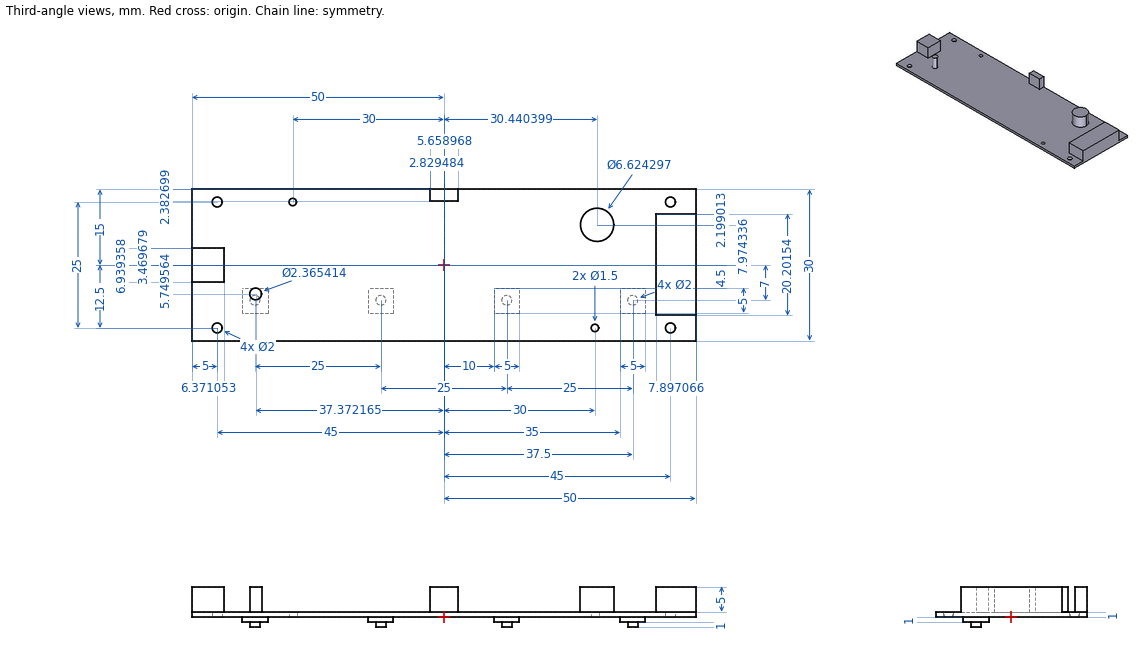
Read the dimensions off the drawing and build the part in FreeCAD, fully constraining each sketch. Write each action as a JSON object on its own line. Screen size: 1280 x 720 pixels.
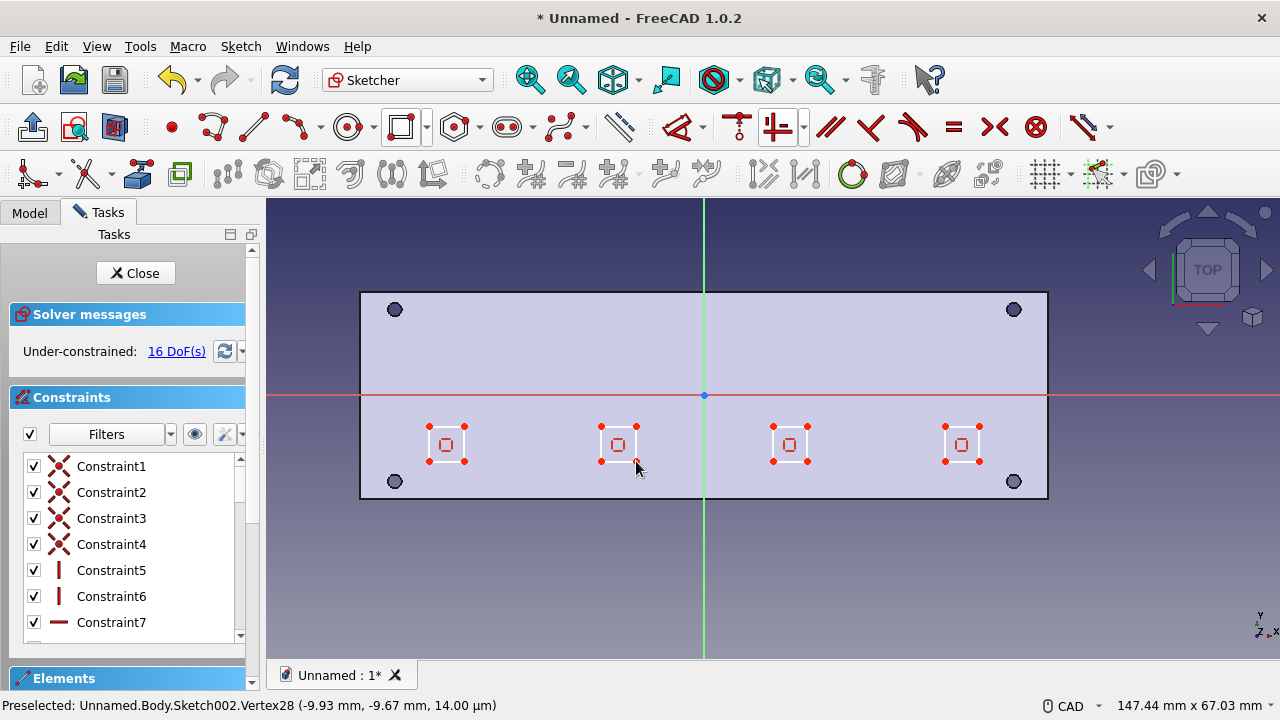
{"action": "left_click", "coordinate": [979, 427]}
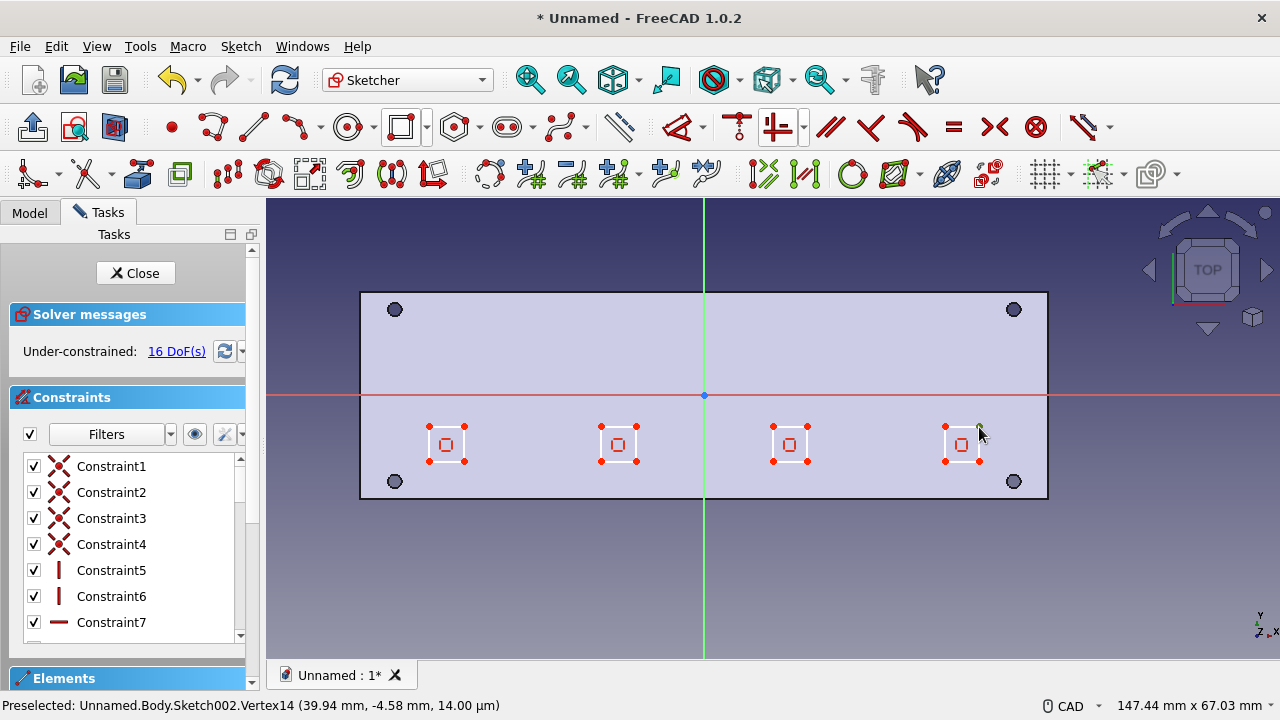
{"action": "left_click", "coordinate": [429, 427]}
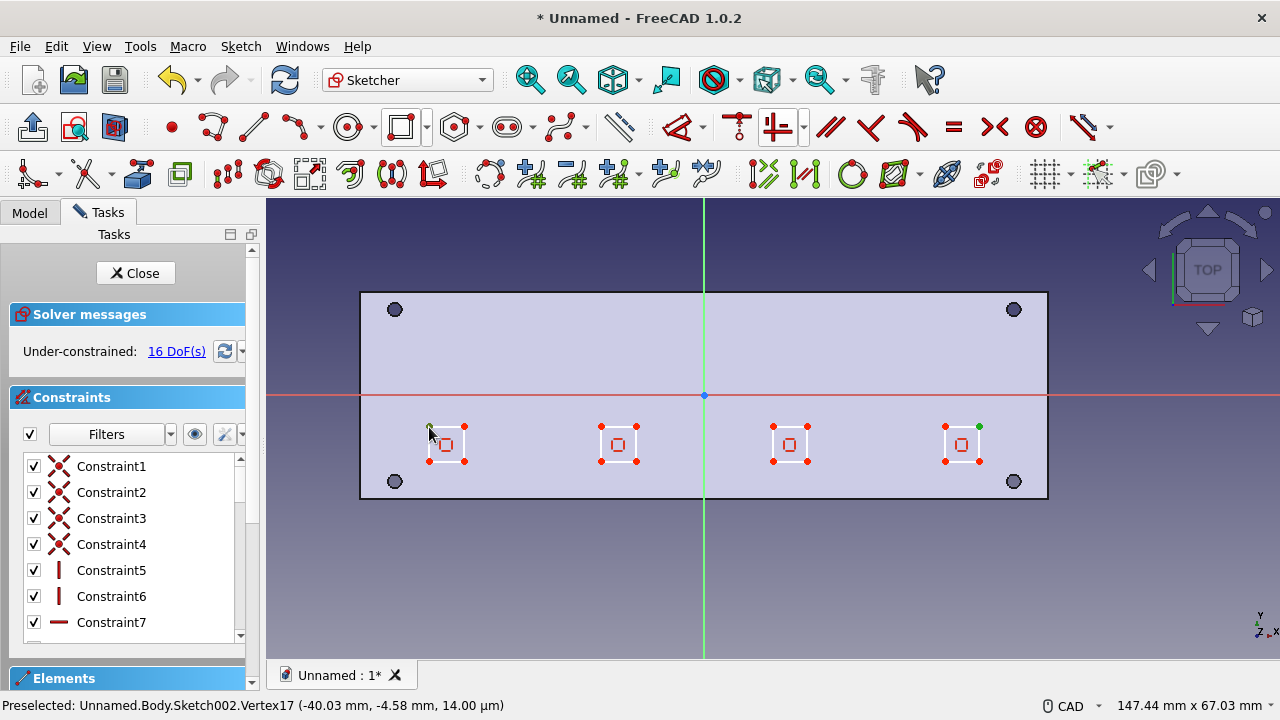
{"action": "left_click", "coordinate": [704, 602]}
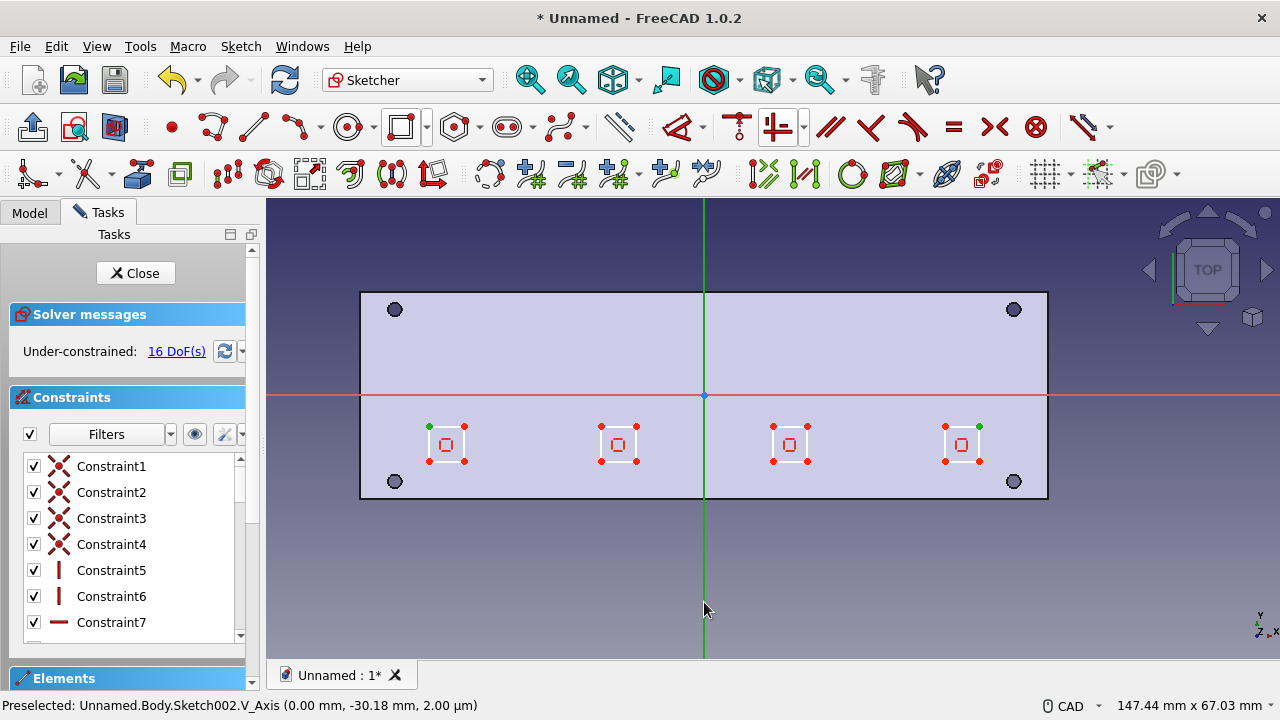
{"action": "key", "text": "s"}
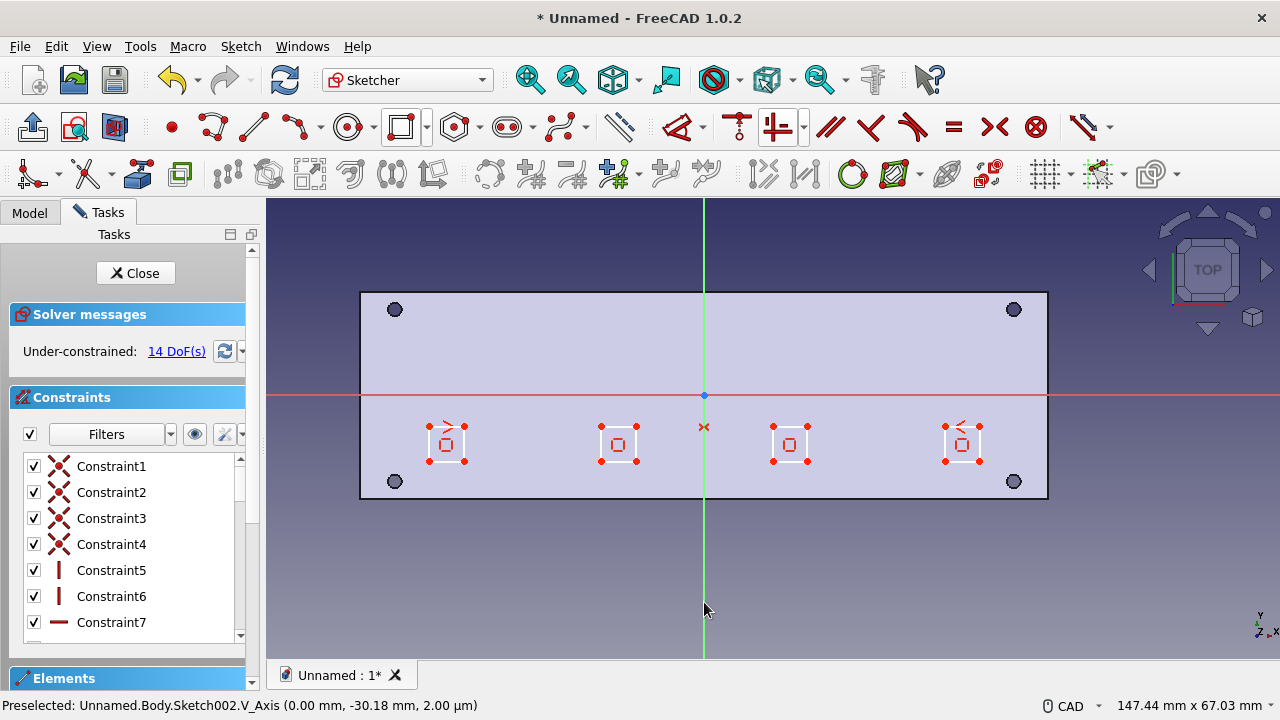
{"action": "left_click", "coordinate": [945, 462]}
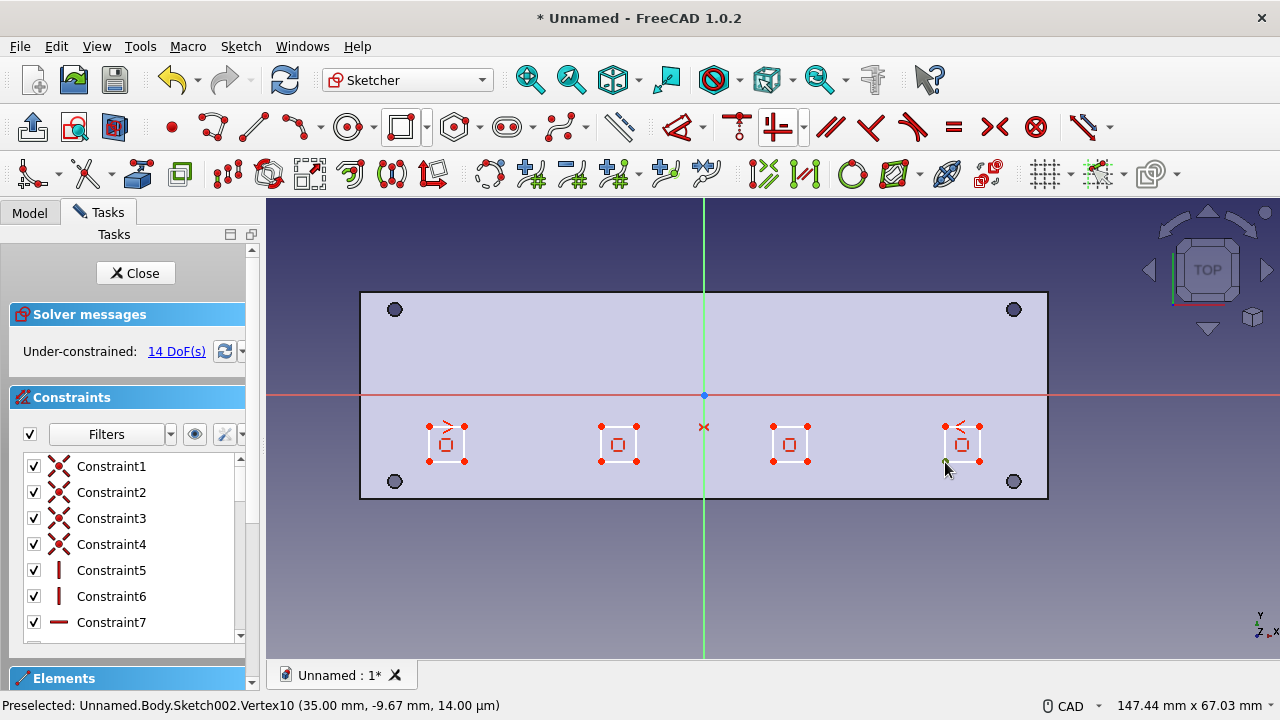
{"action": "left_click", "coordinate": [464, 462]}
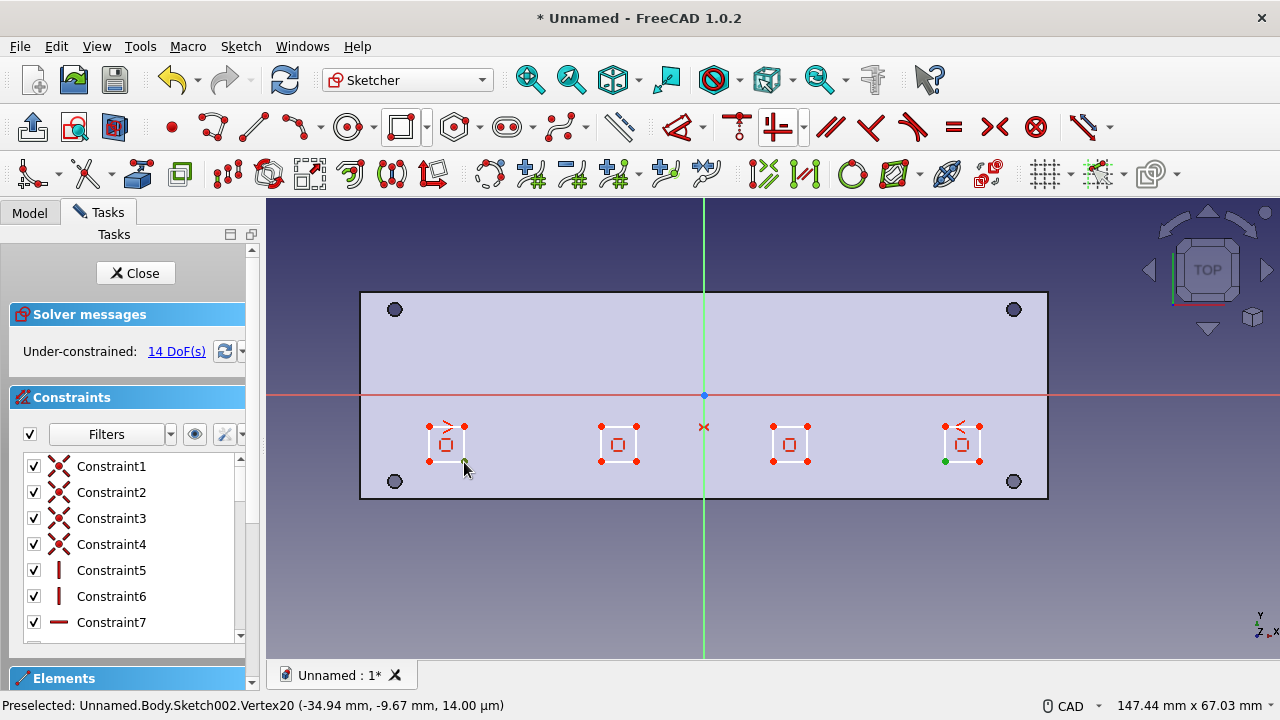
{"action": "left_click", "coordinate": [704, 602]}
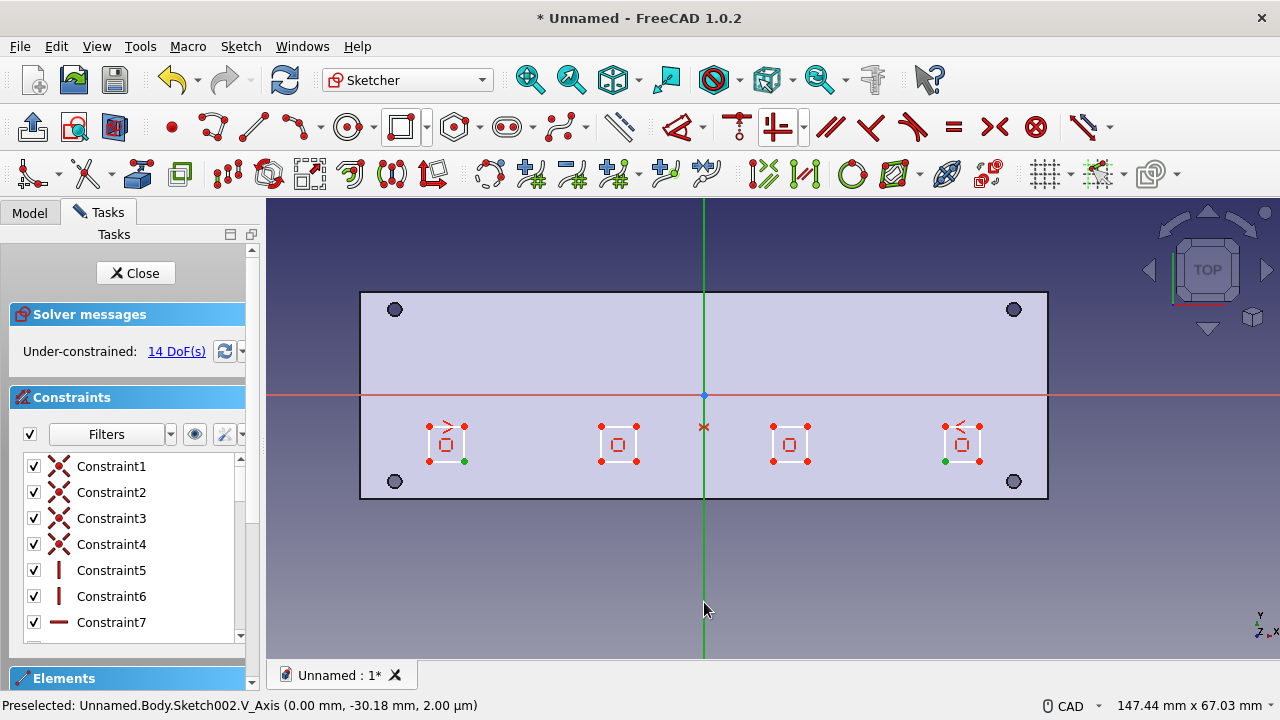
{"action": "left_click", "coordinate": [995, 128]}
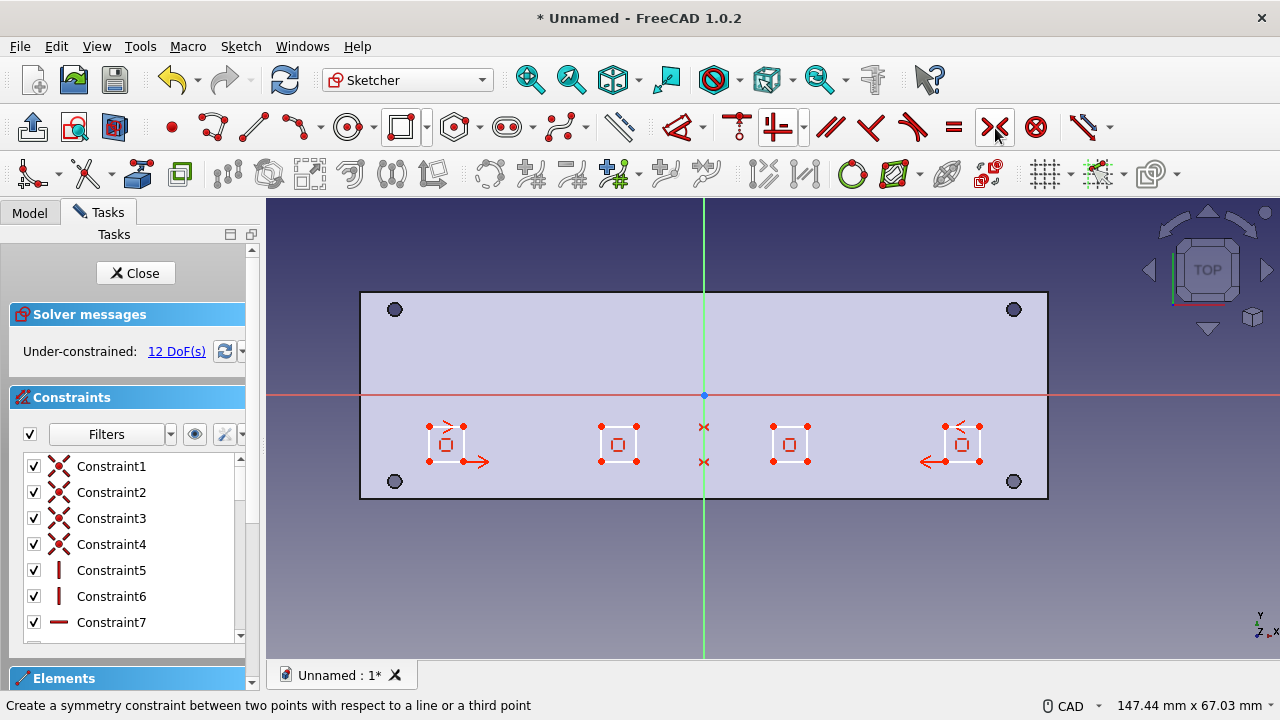
{"action": "left_click", "coordinate": [807, 427]}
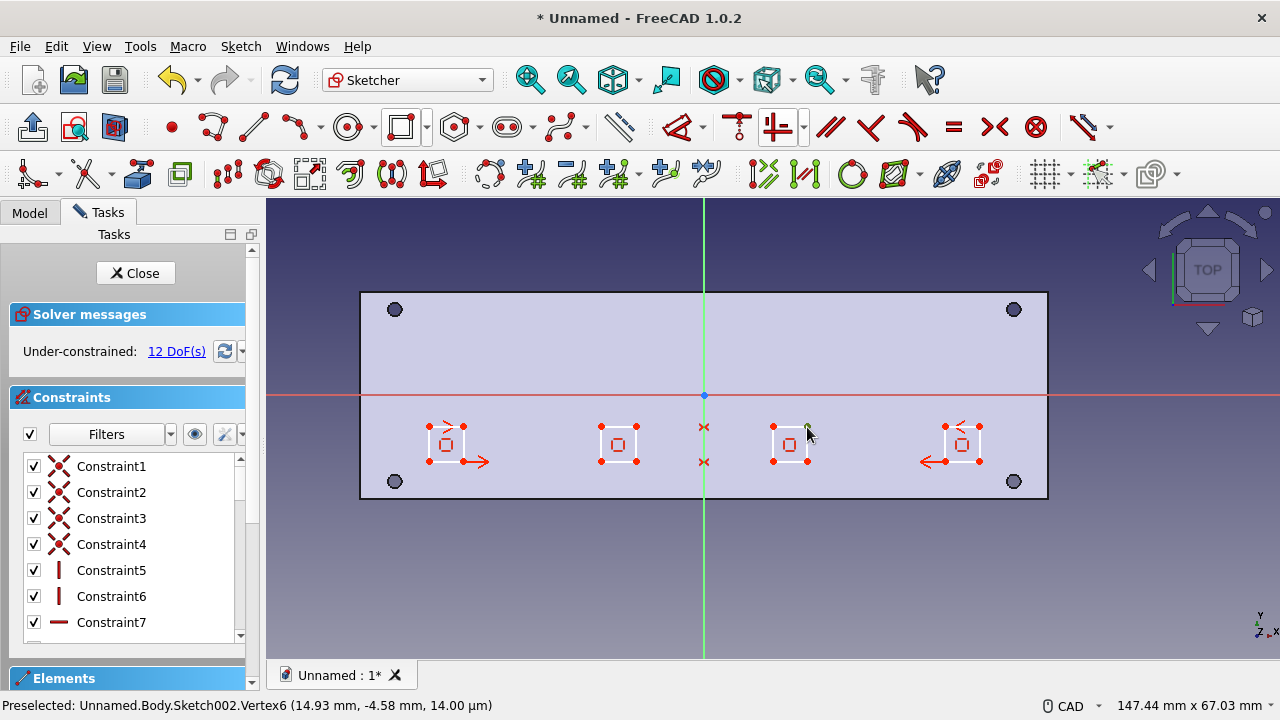
{"action": "left_click", "coordinate": [601, 427]}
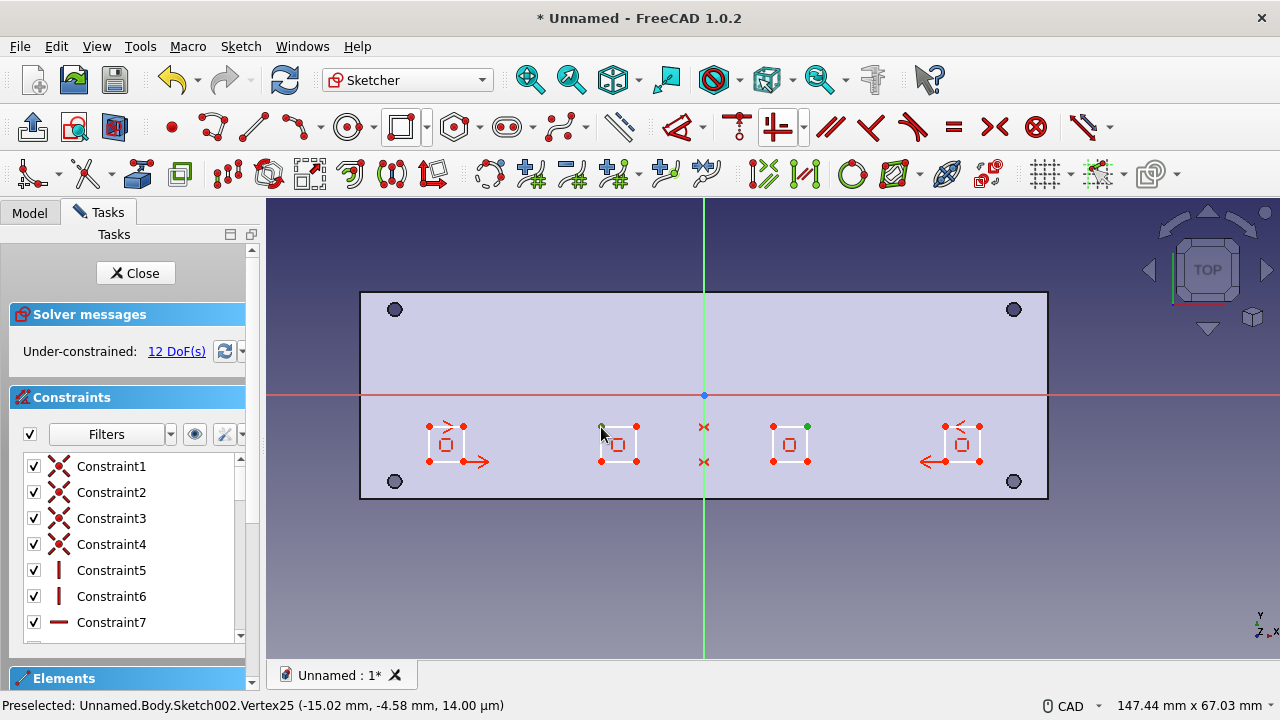
{"action": "left_click", "coordinate": [704, 602]}